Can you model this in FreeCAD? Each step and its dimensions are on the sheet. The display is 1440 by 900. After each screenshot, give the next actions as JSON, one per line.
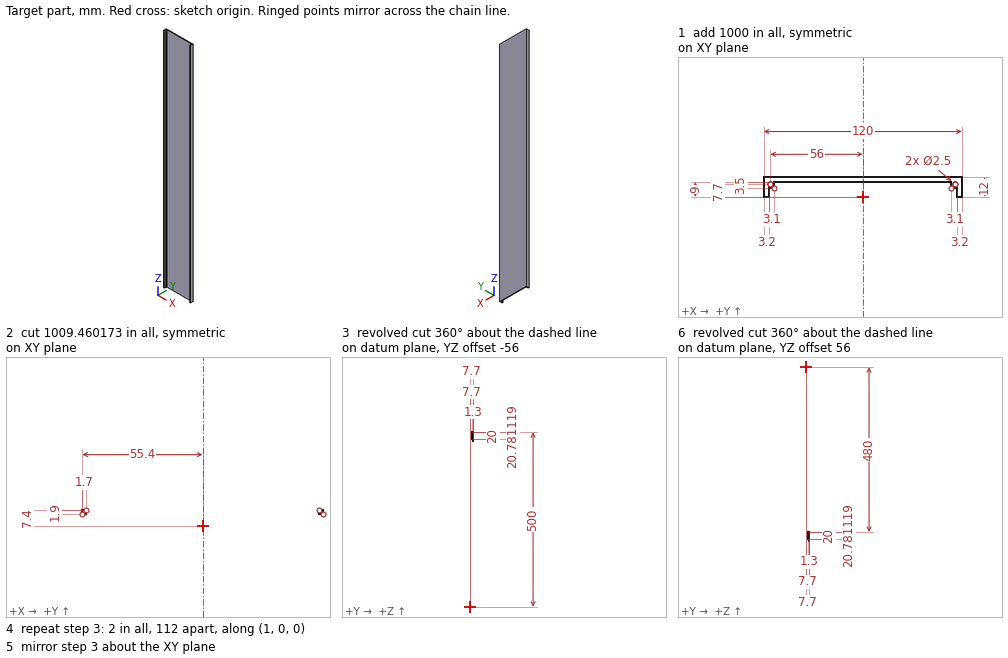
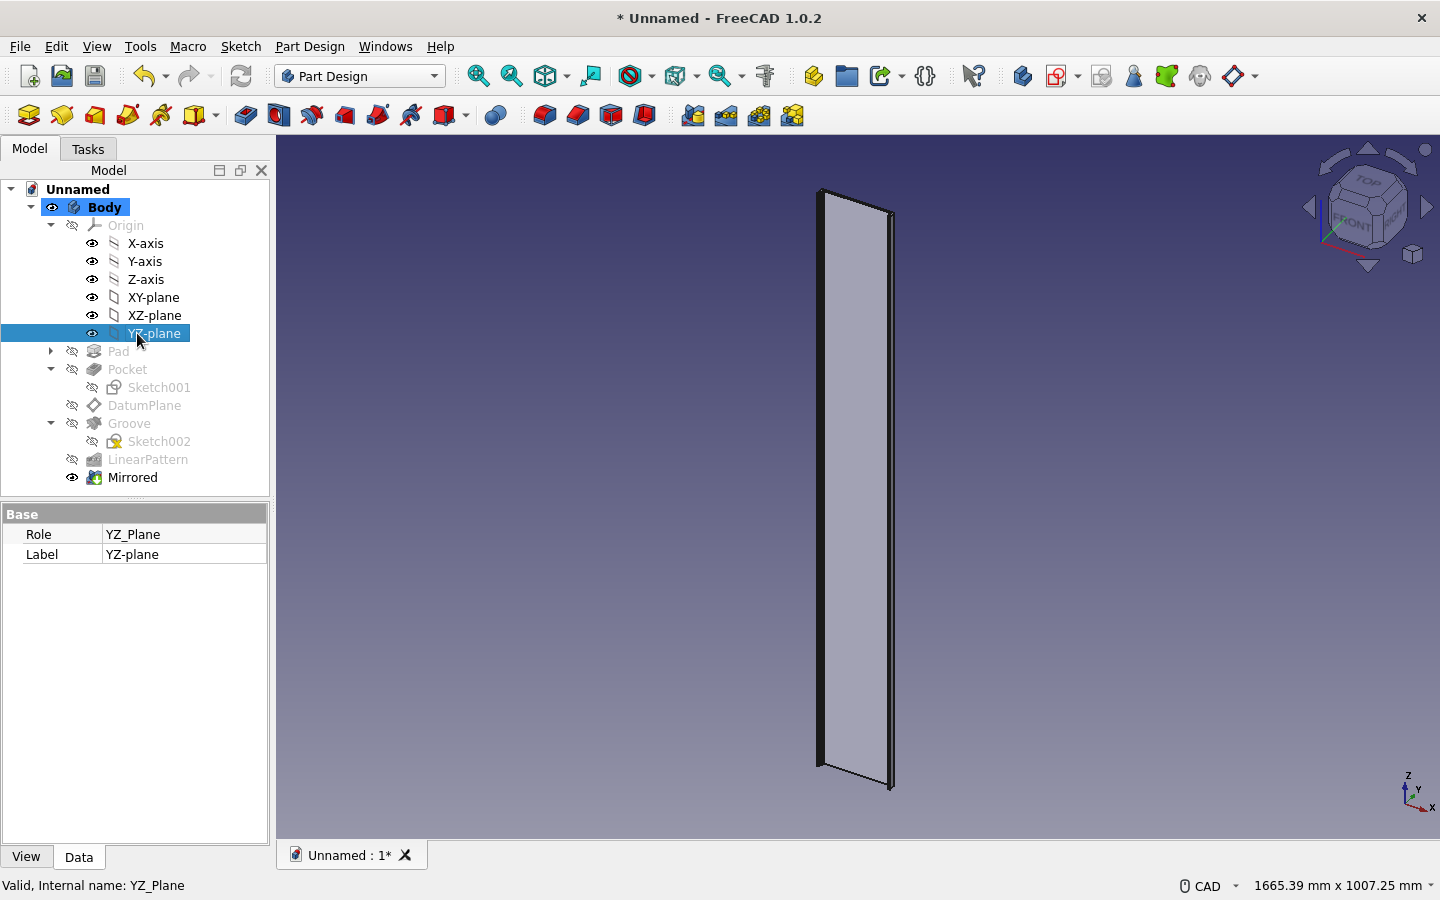
{"action": "left_click", "coordinate": [1232, 76]}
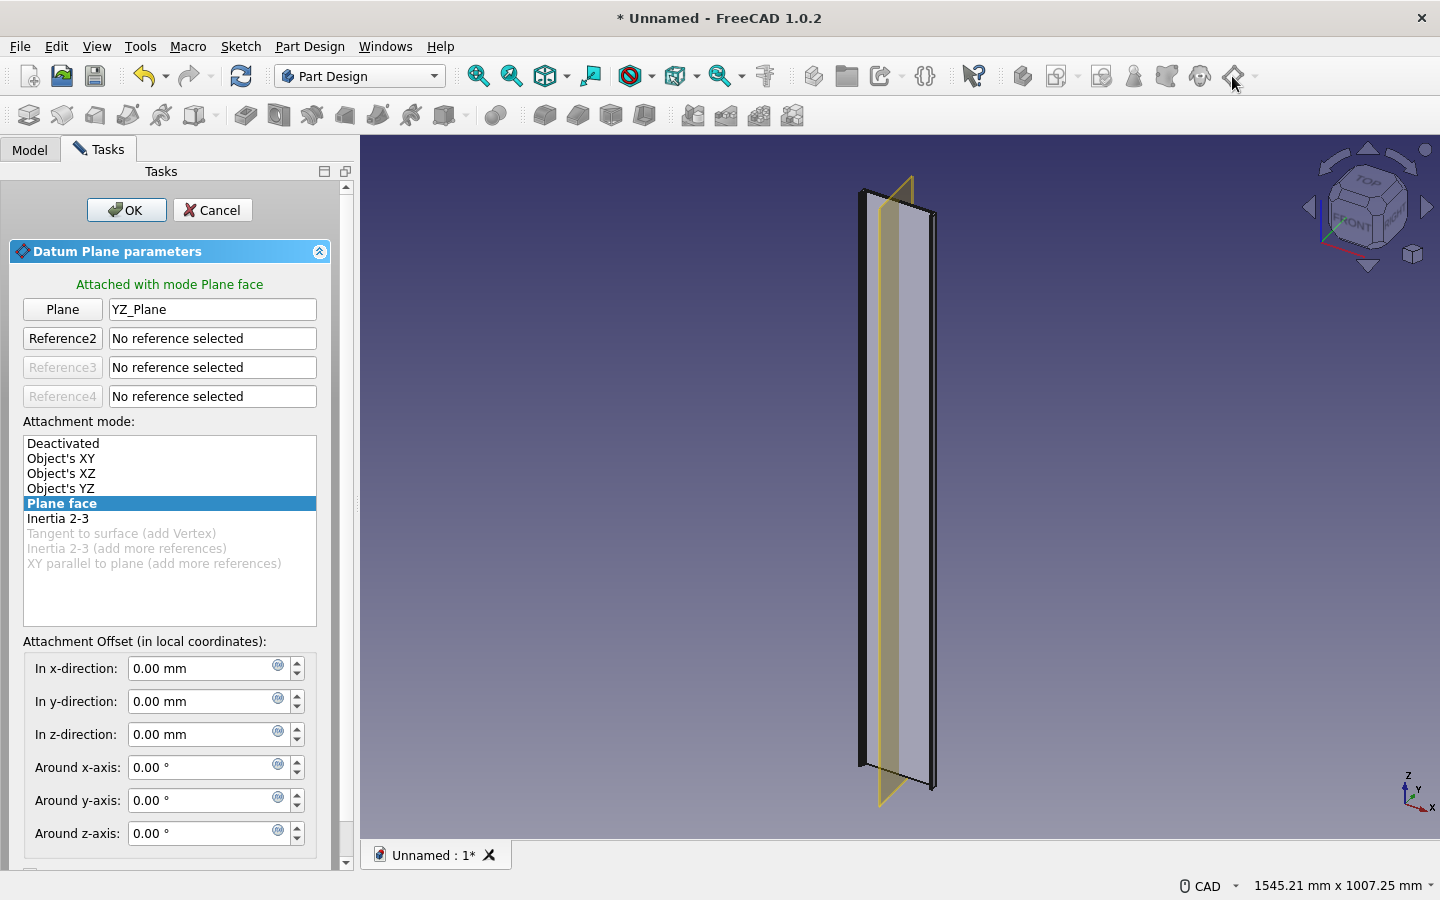
{"action": "triple_click", "coordinate": [210, 734]}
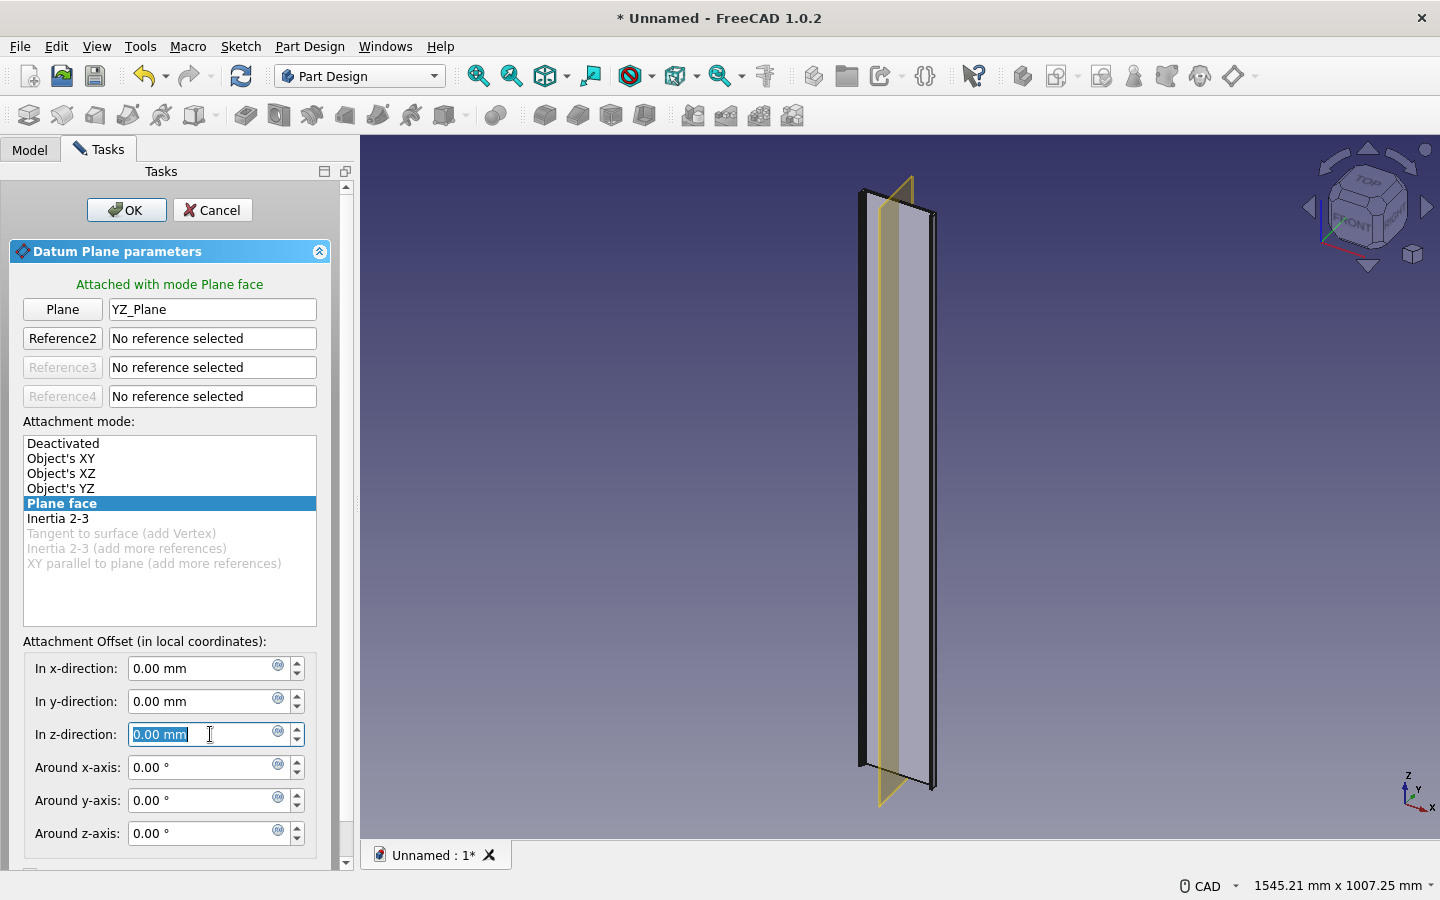
{"action": "type", "text": "56"}
{"action": "key", "text": "Tab"}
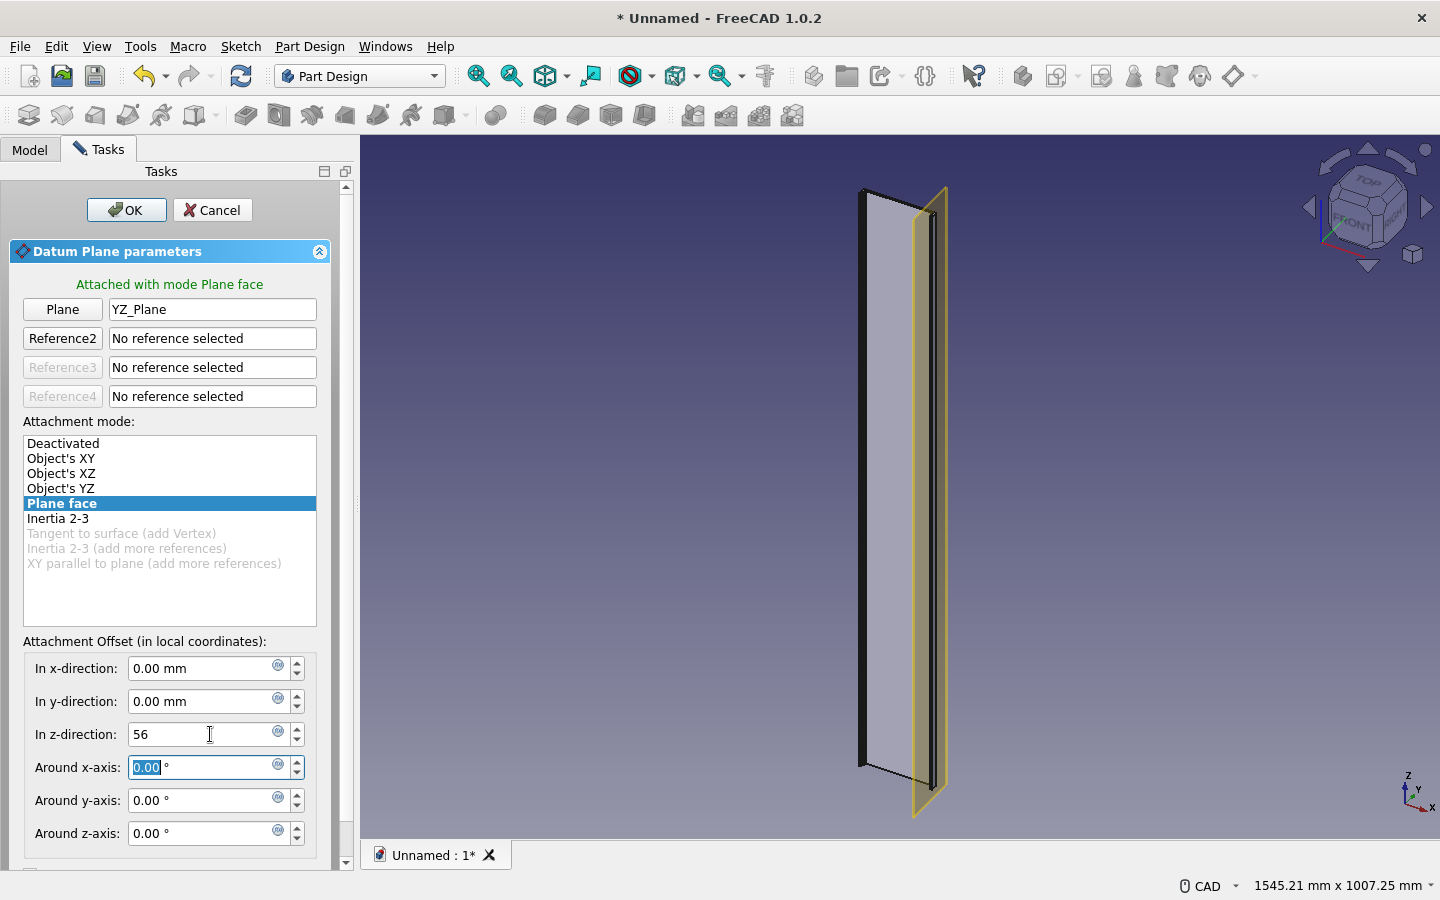
{"action": "left_click", "coordinate": [127, 210]}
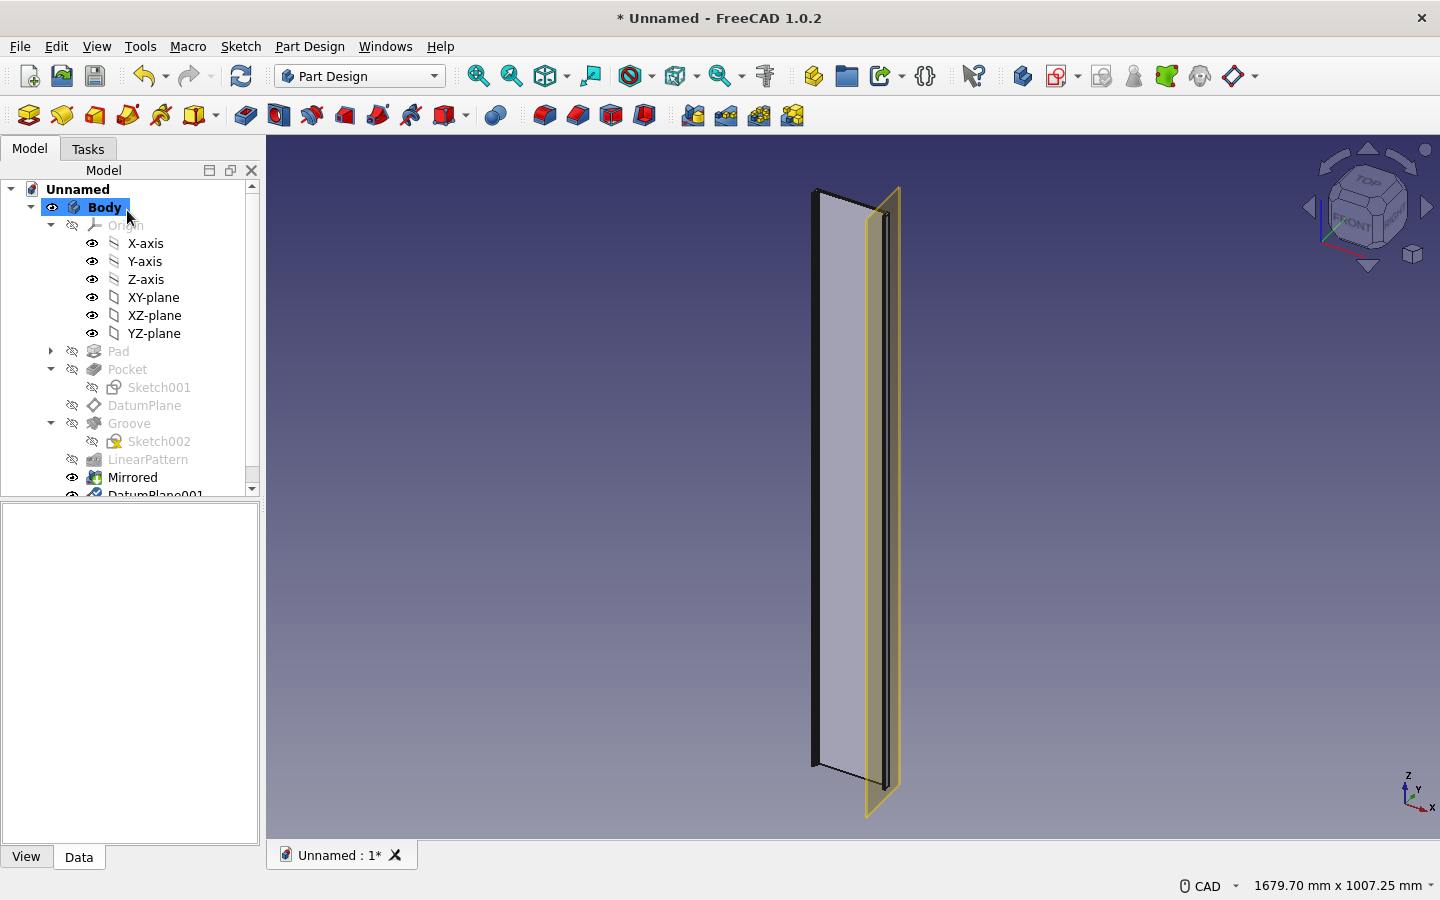
{"action": "left_click", "coordinate": [117, 495]}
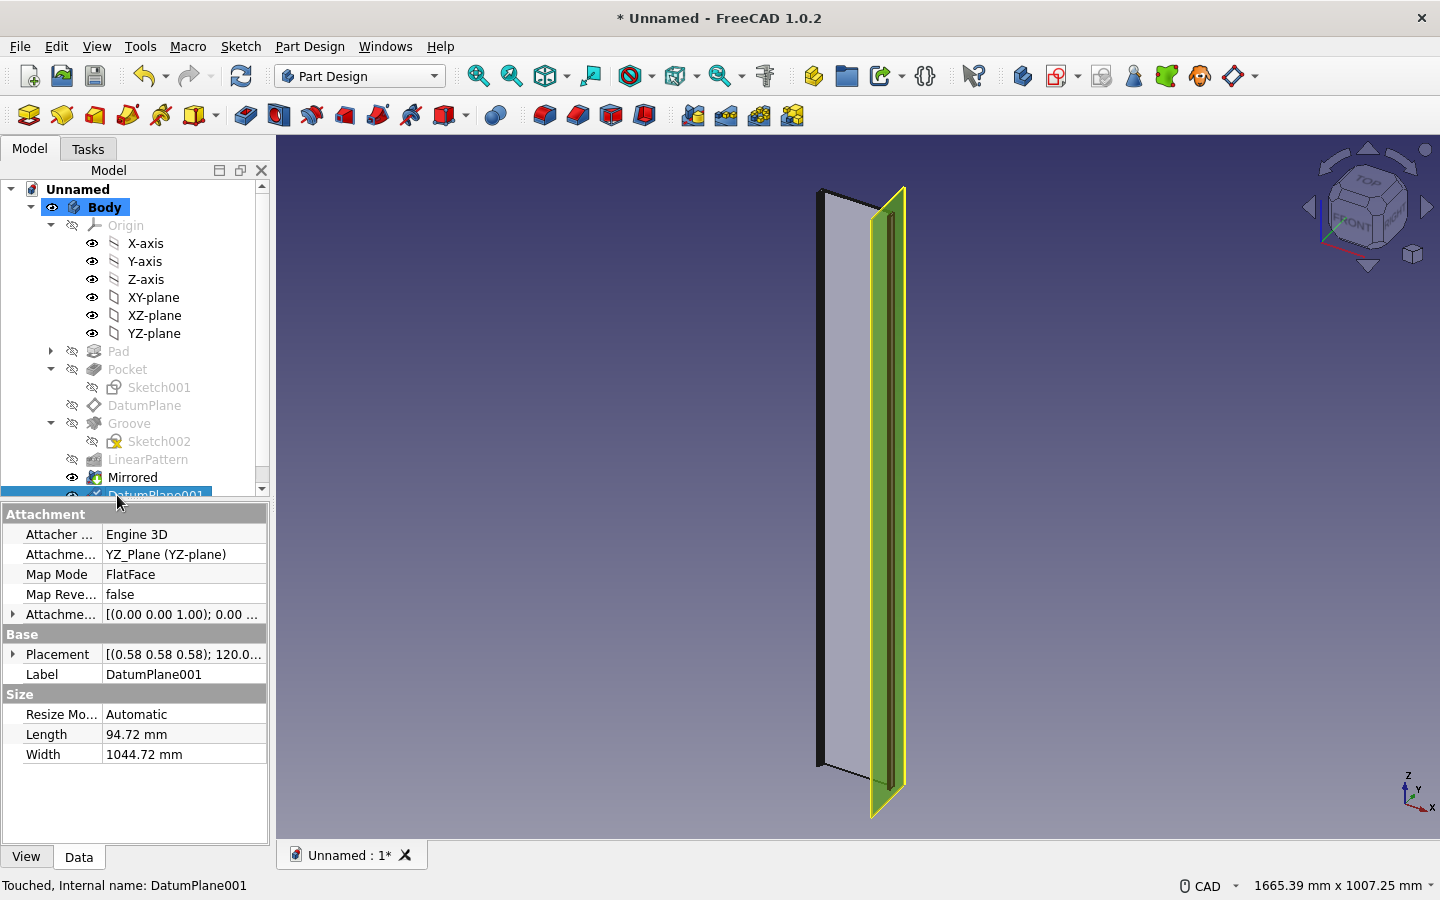
{"action": "left_click", "coordinate": [1056, 76]}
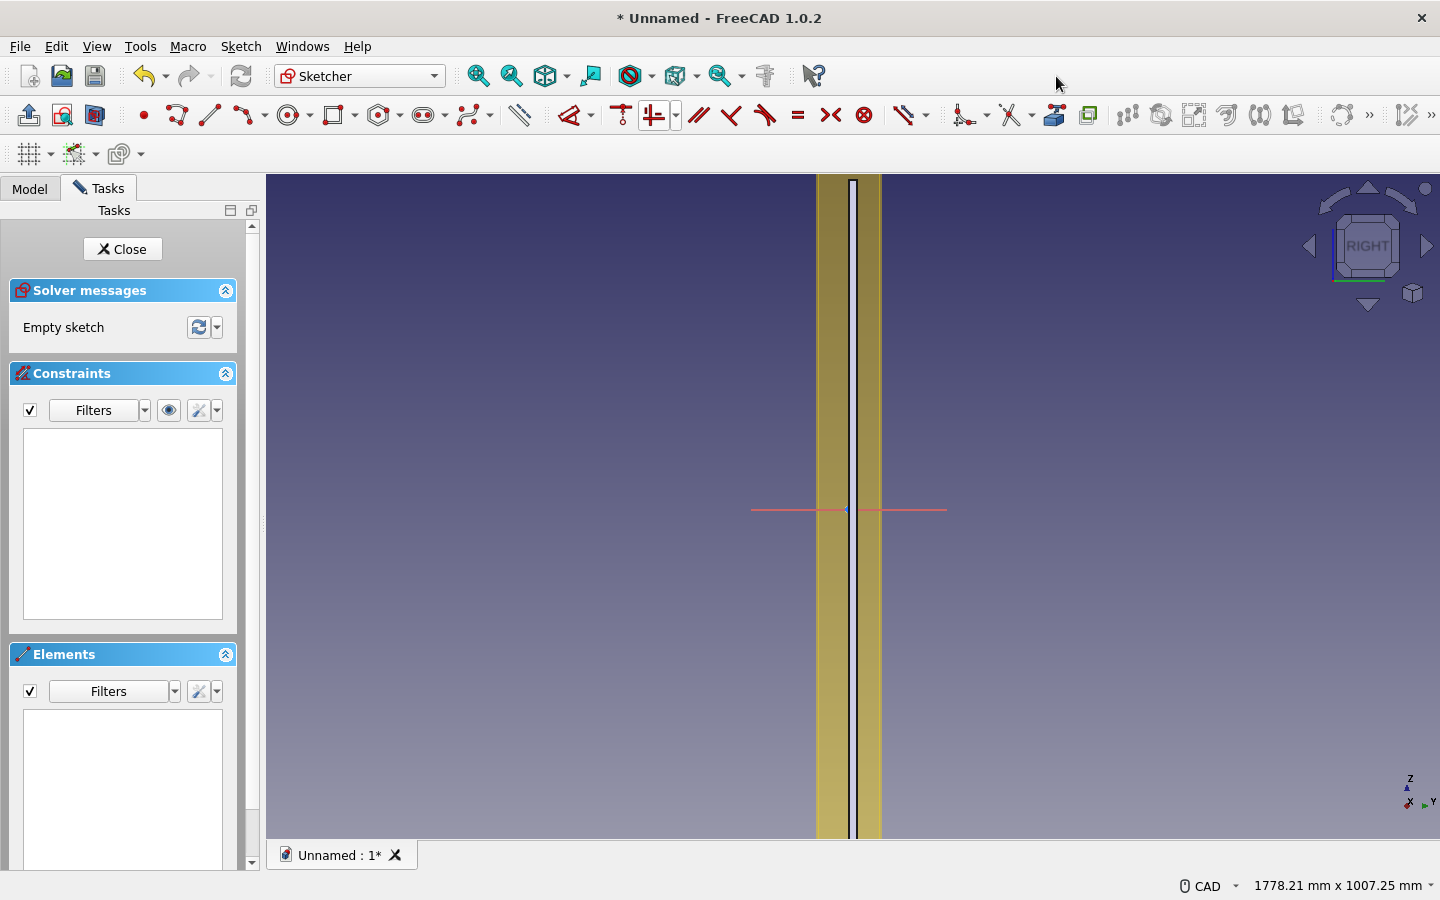
{"action": "key", "text": "q s"}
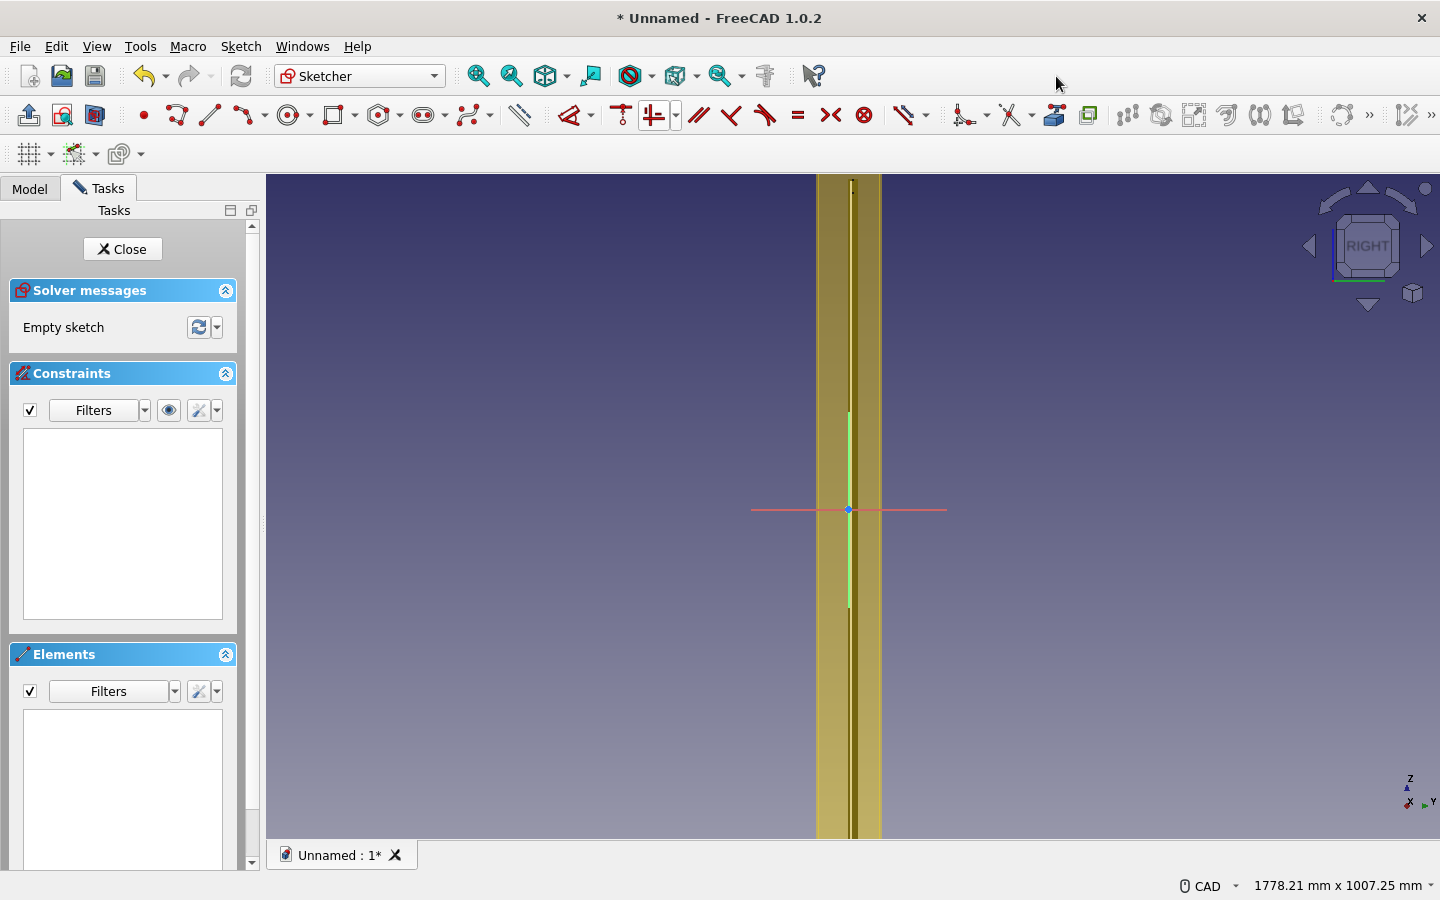
{"action": "scroll", "coordinate": [784, 506], "scroll_direction": "down", "scroll_amount": 5}